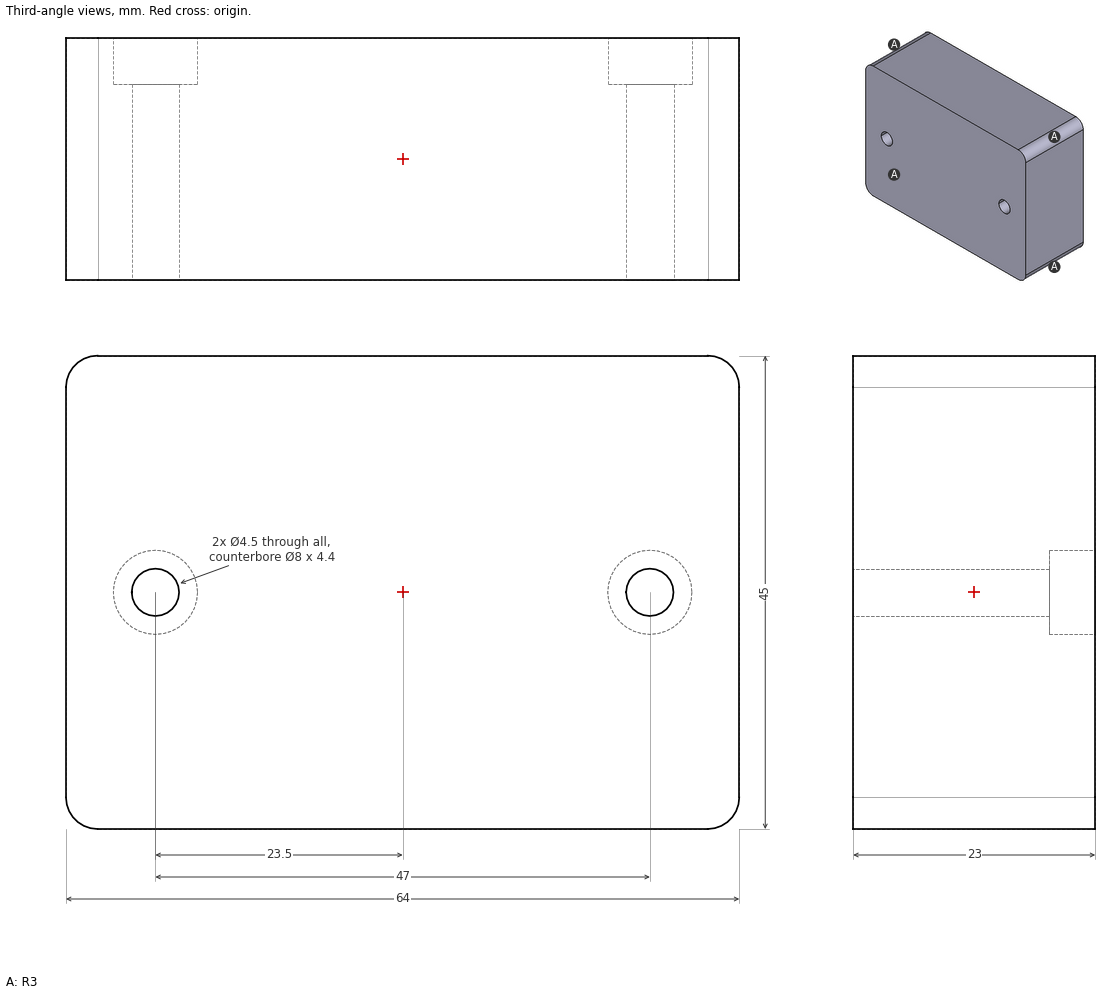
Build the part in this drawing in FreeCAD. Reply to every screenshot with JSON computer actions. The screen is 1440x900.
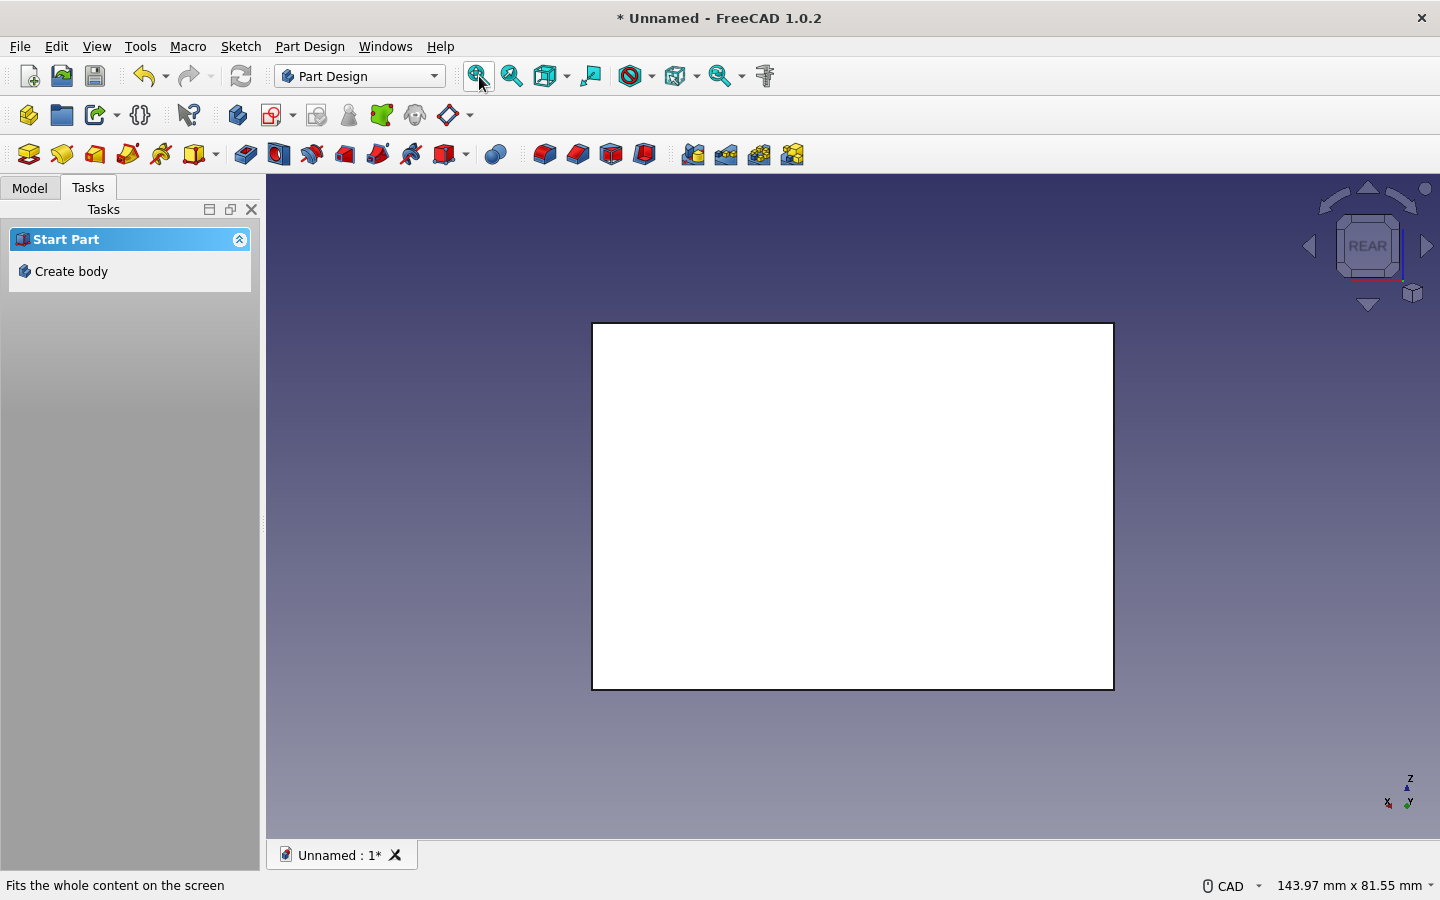
{"action": "left_click", "coordinate": [778, 506]}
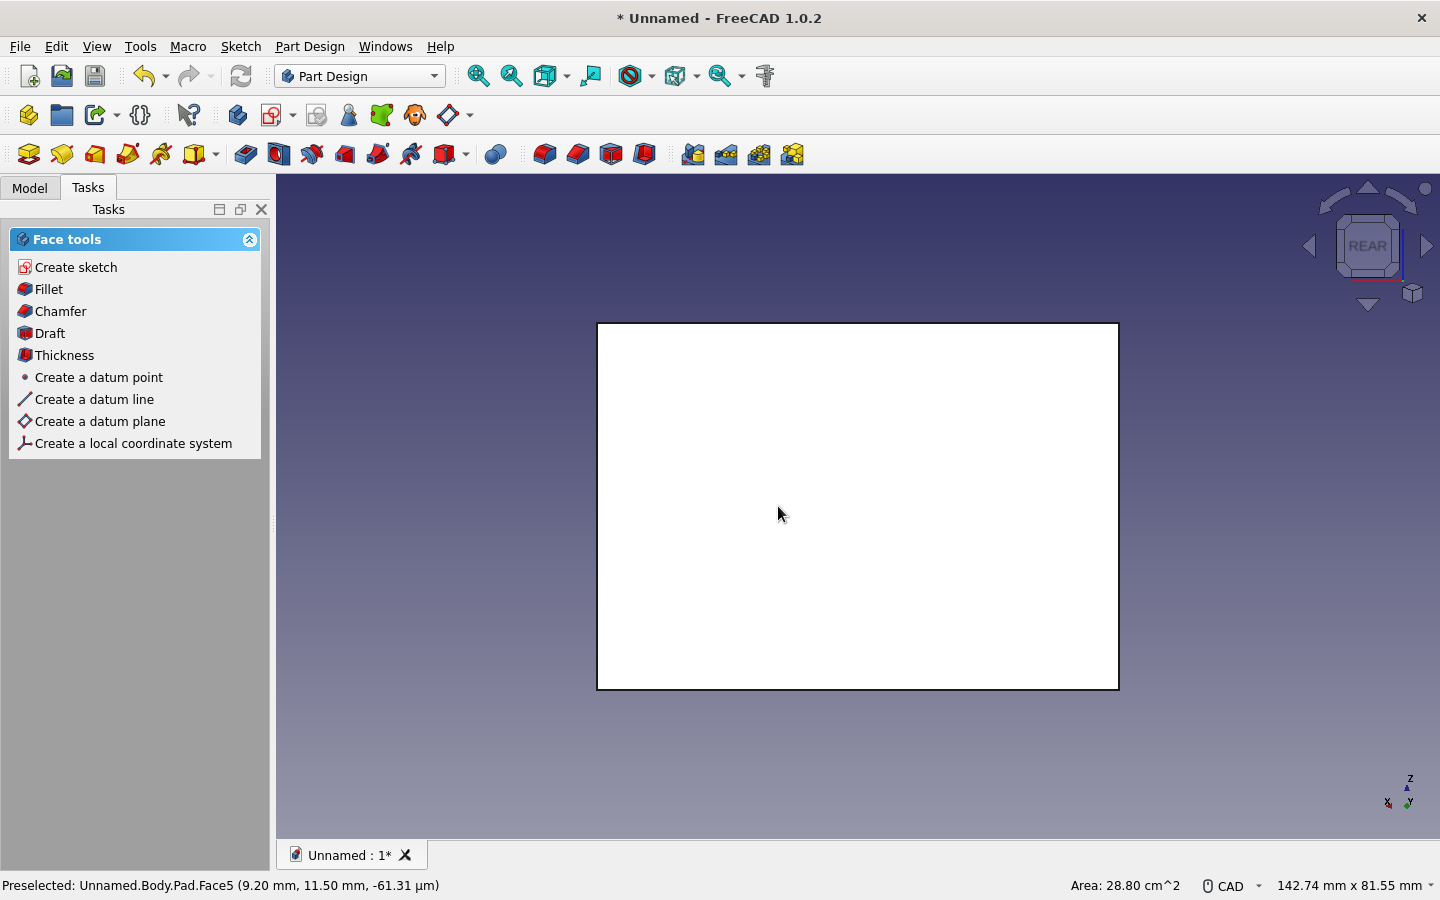
{"action": "left_click", "coordinate": [270, 116]}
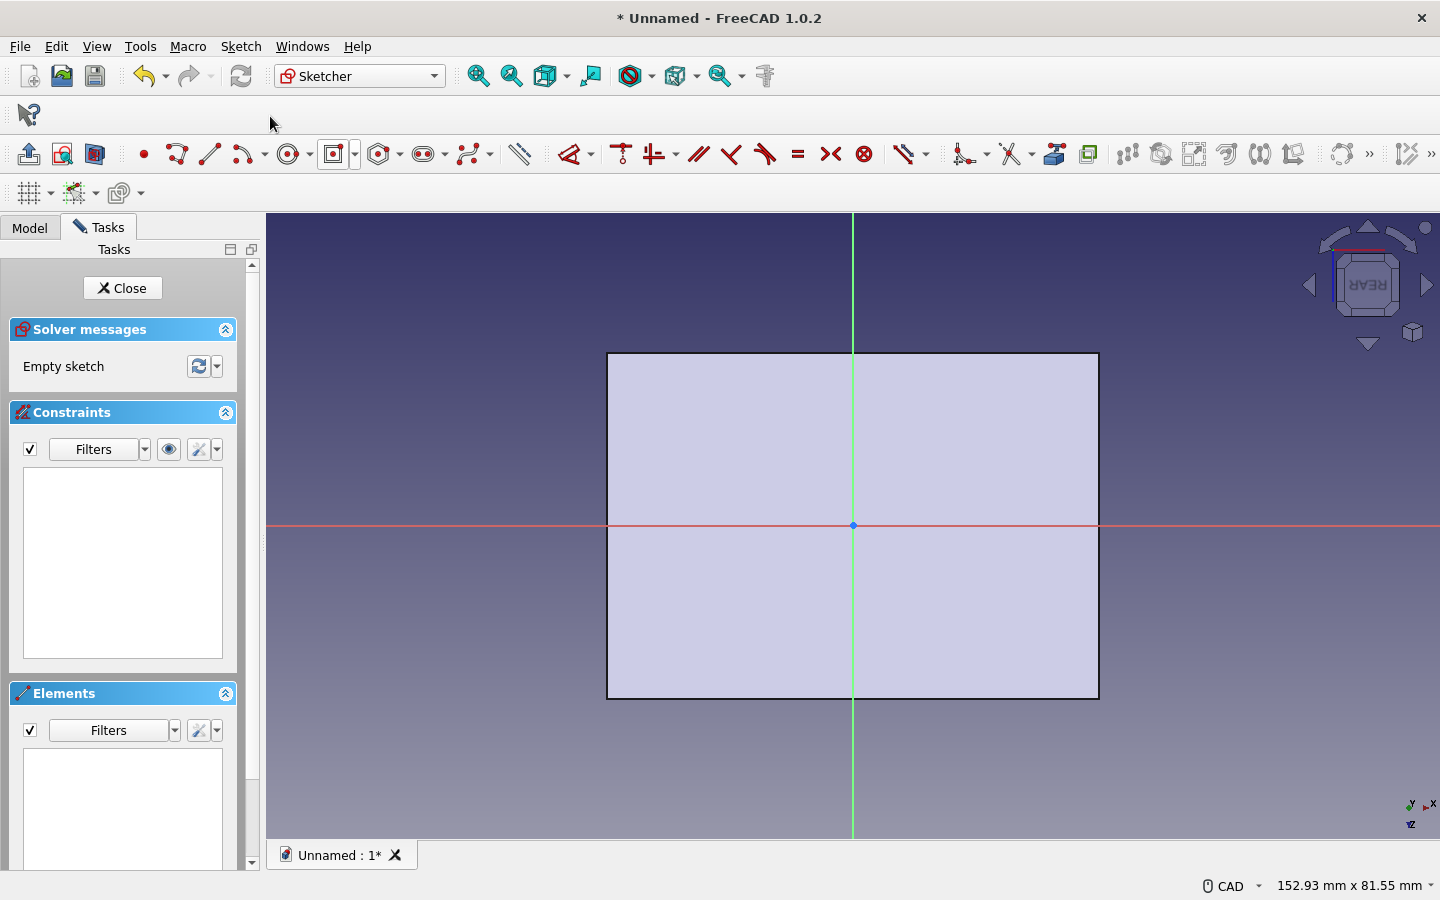
{"action": "scroll", "coordinate": [936, 526], "scroll_direction": "up", "scroll_amount": 3}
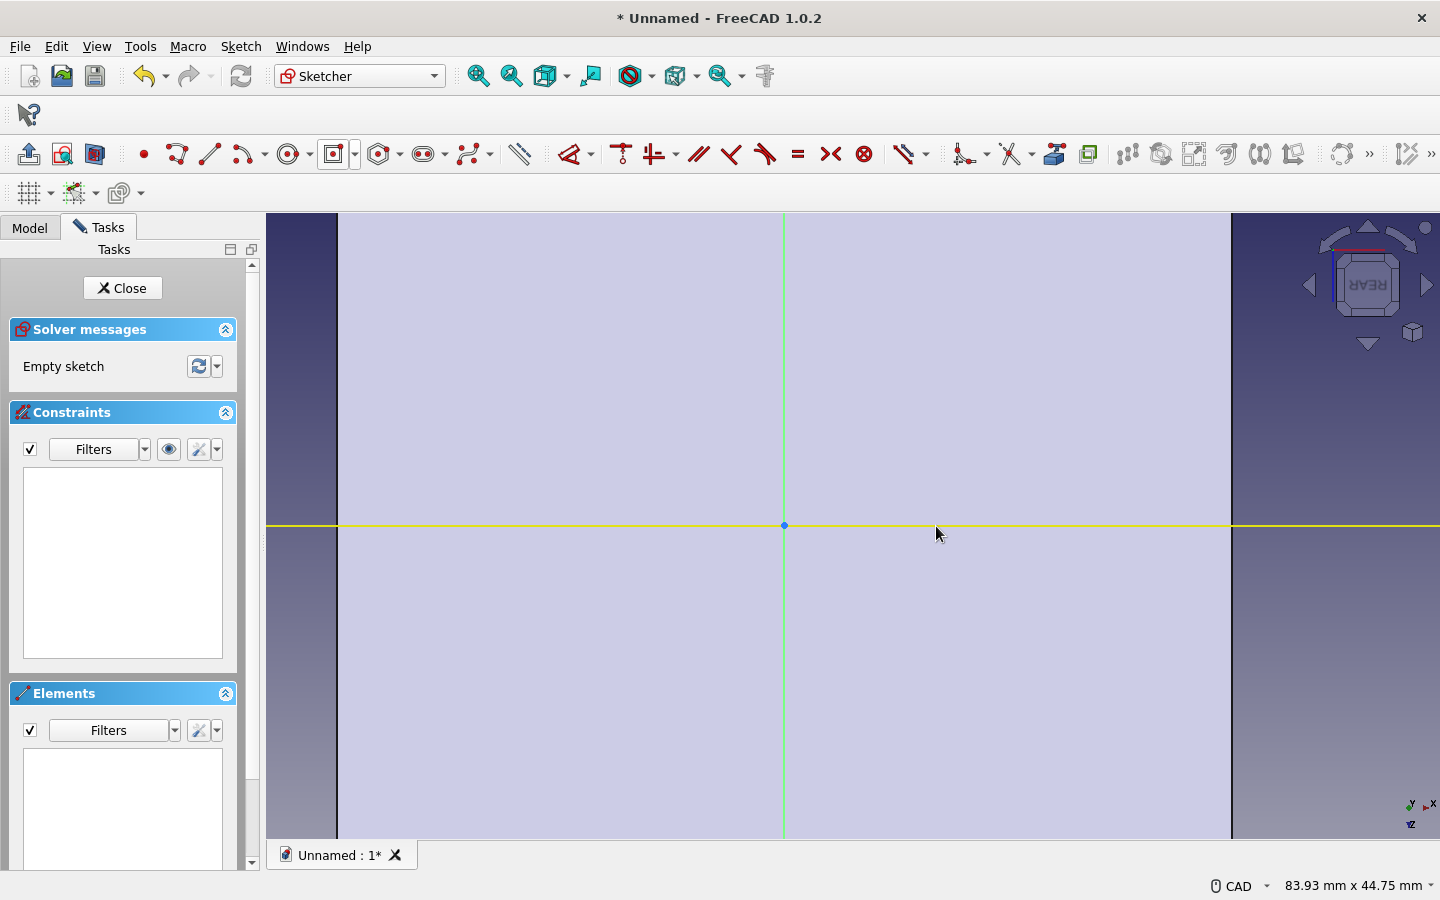
{"action": "left_click", "coordinate": [288, 154]}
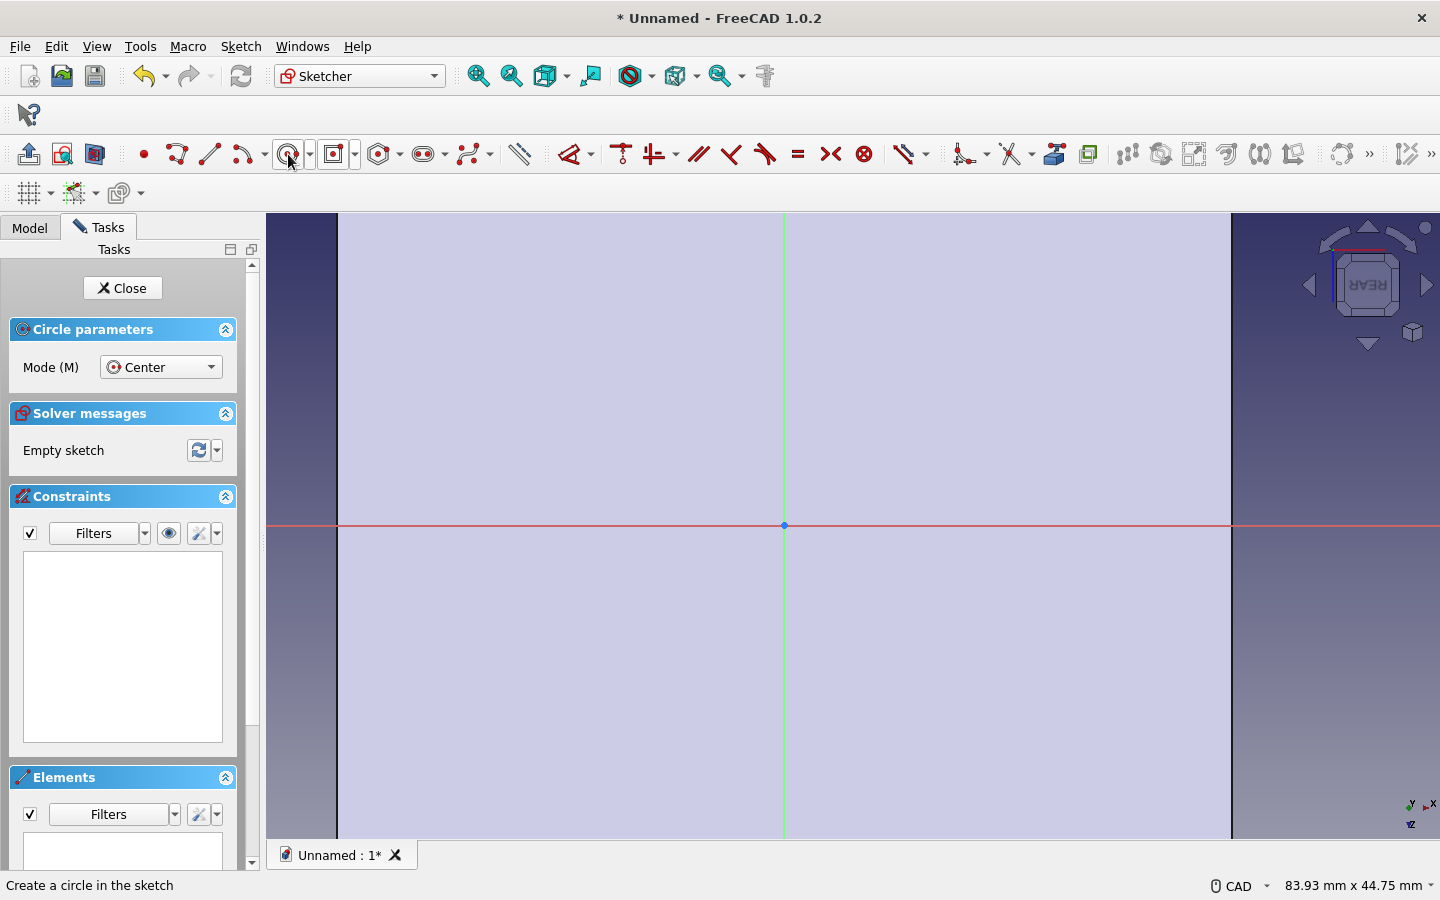
{"action": "left_click", "coordinate": [456, 526]}
{"action": "left_click", "coordinate": [478, 503]}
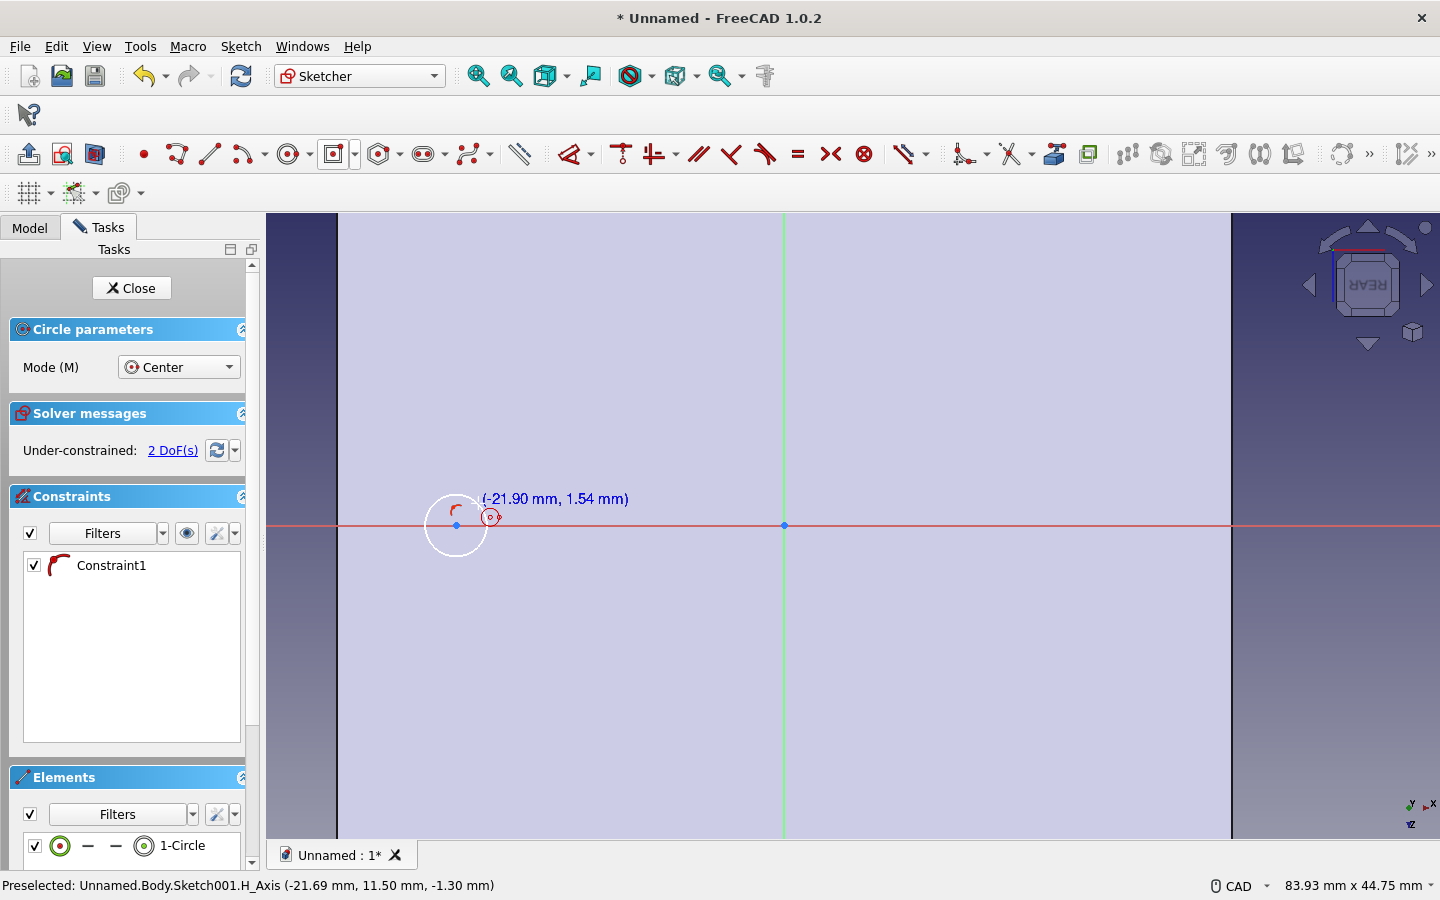
{"action": "left_click", "coordinate": [1113, 526]}
{"action": "left_click", "coordinate": [1135, 503]}
{"action": "key", "text": "Escape"}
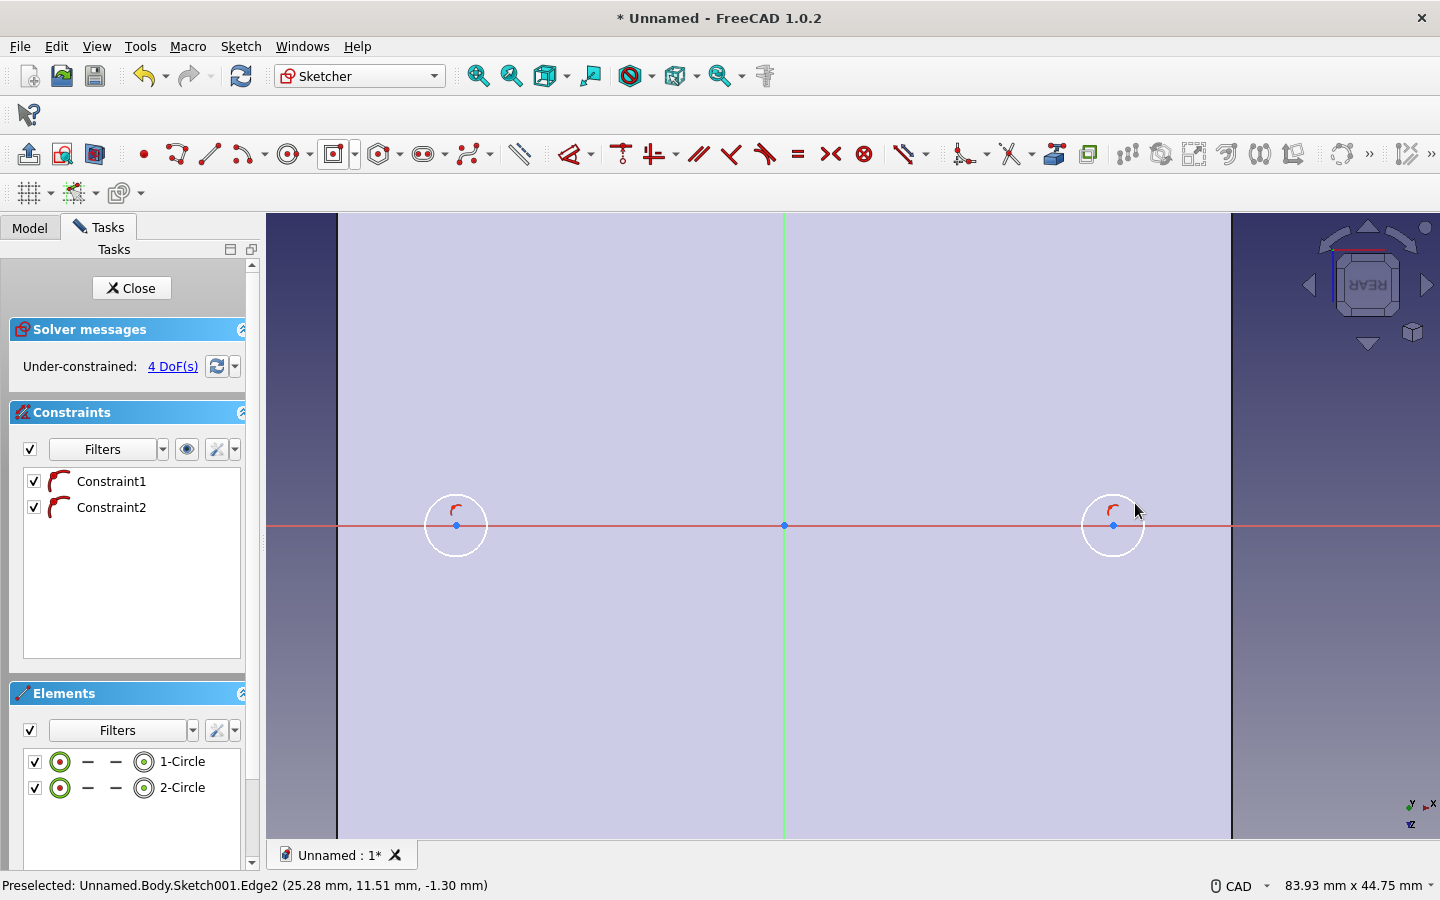
{"action": "left_click", "coordinate": [478, 504]}